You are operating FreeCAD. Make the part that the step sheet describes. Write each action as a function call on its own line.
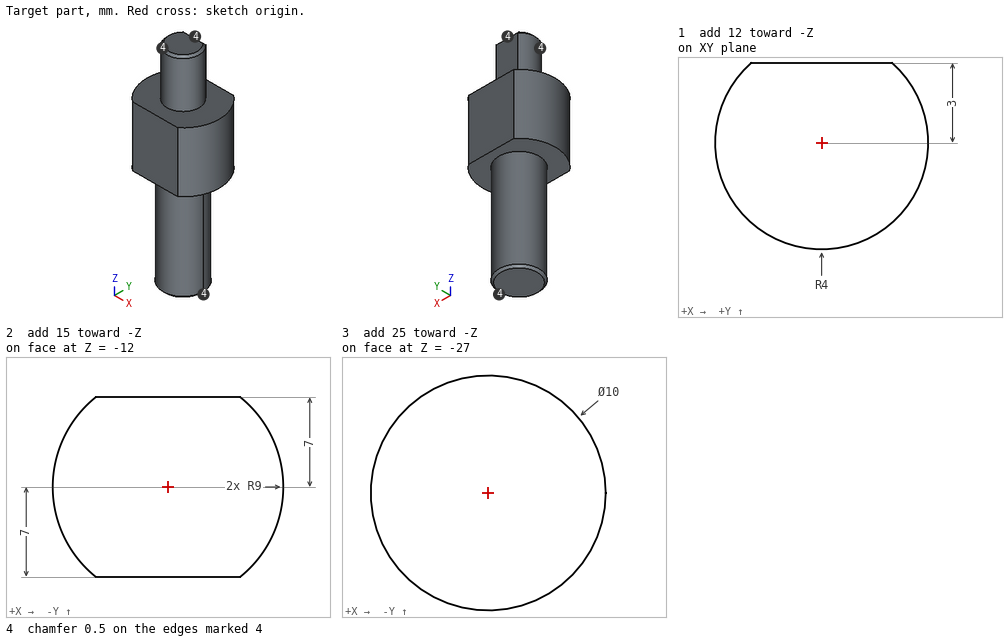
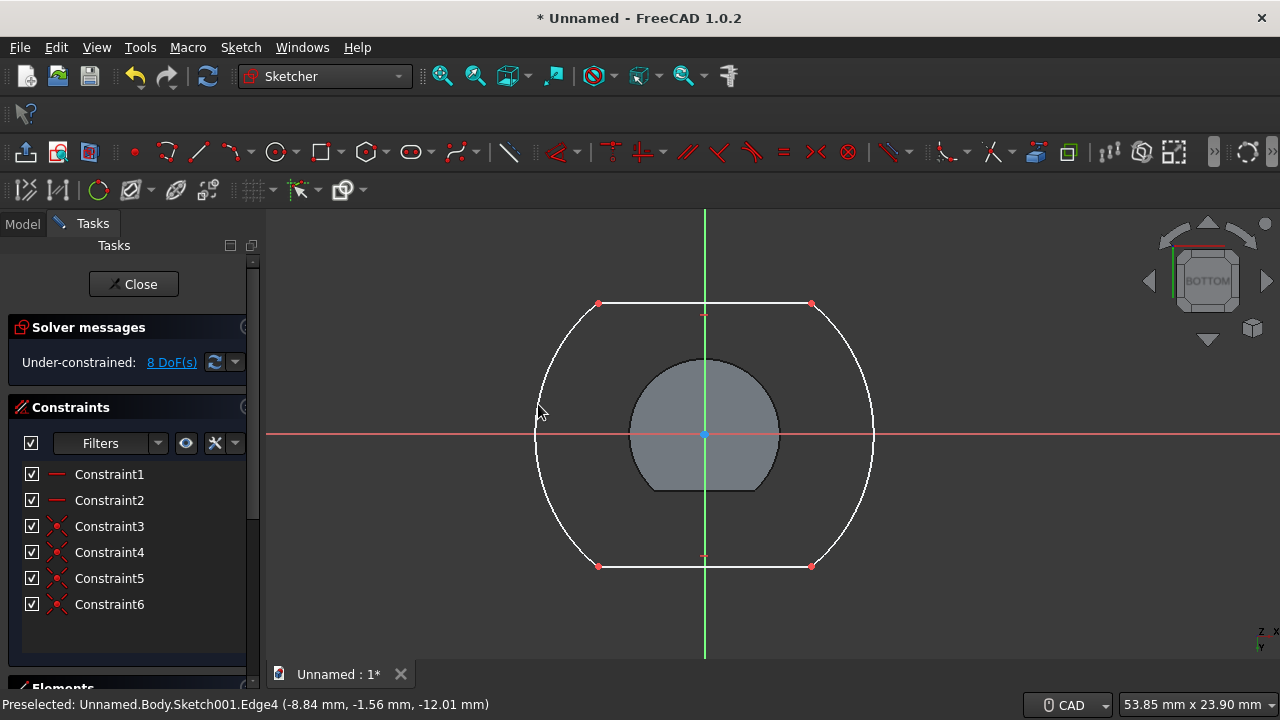
click(863, 494)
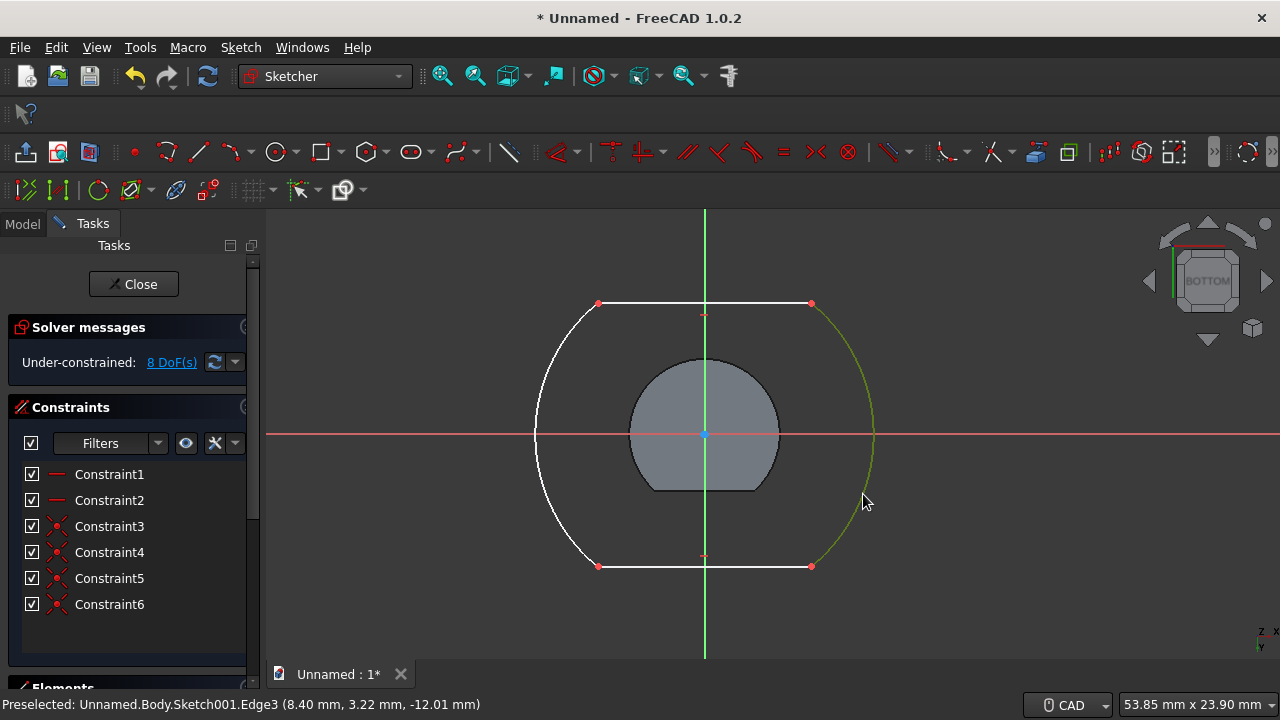
click(546, 376)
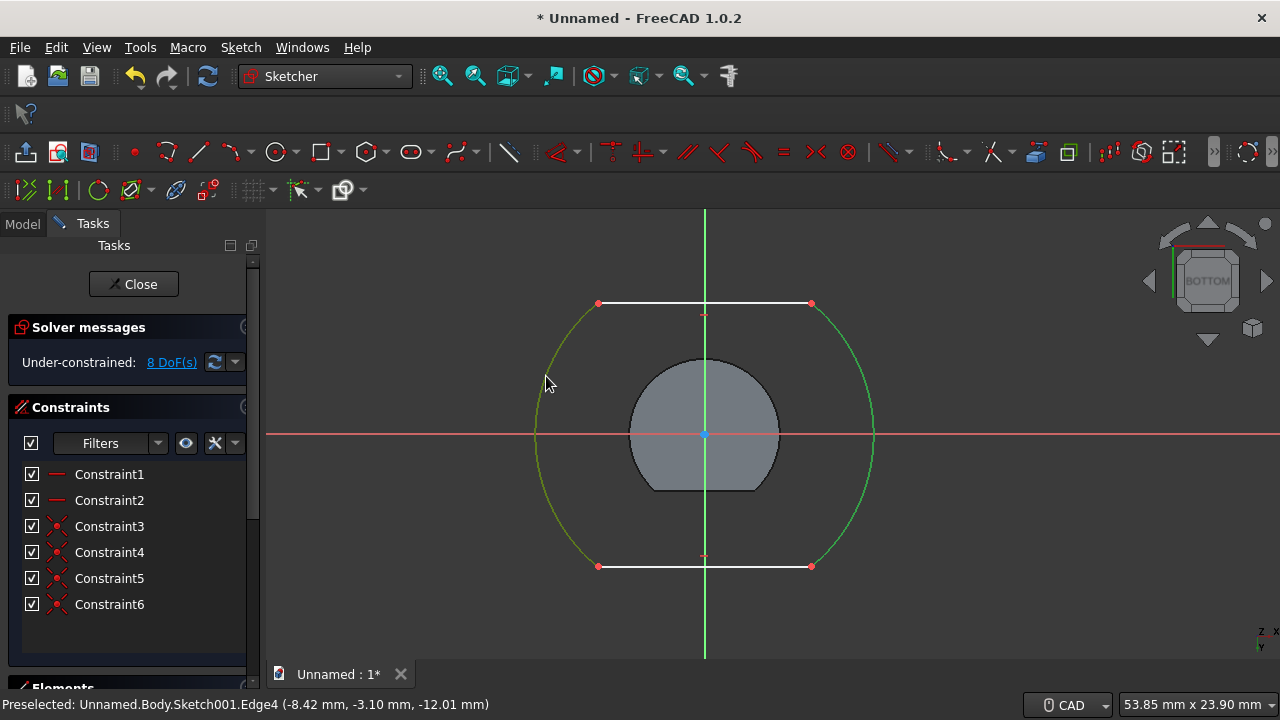
key(c)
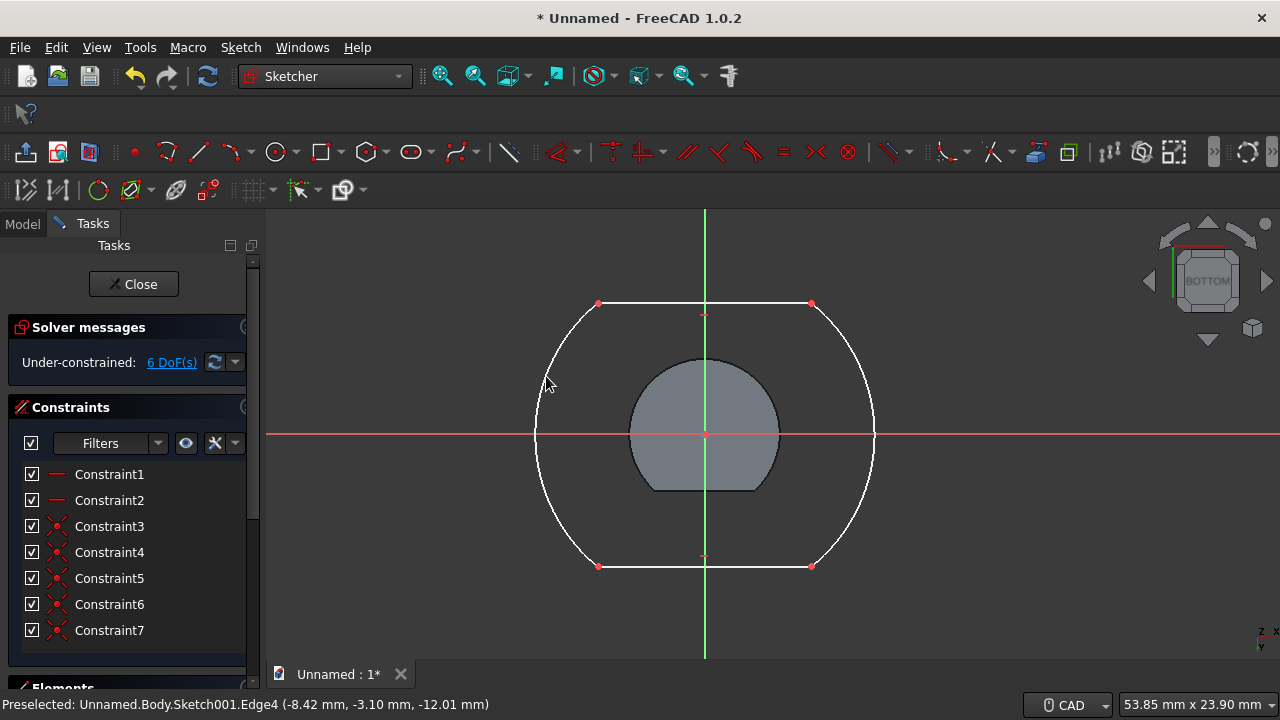
drag(695, 424, 716, 445)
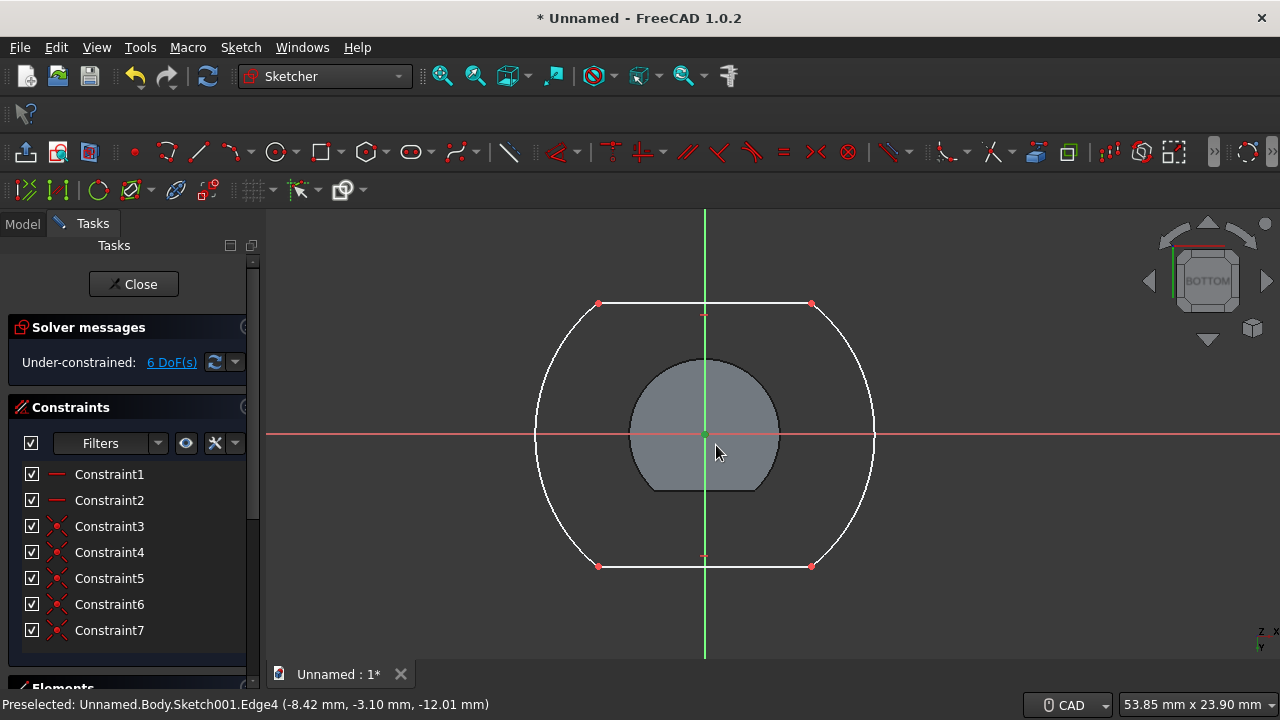
click(612, 152)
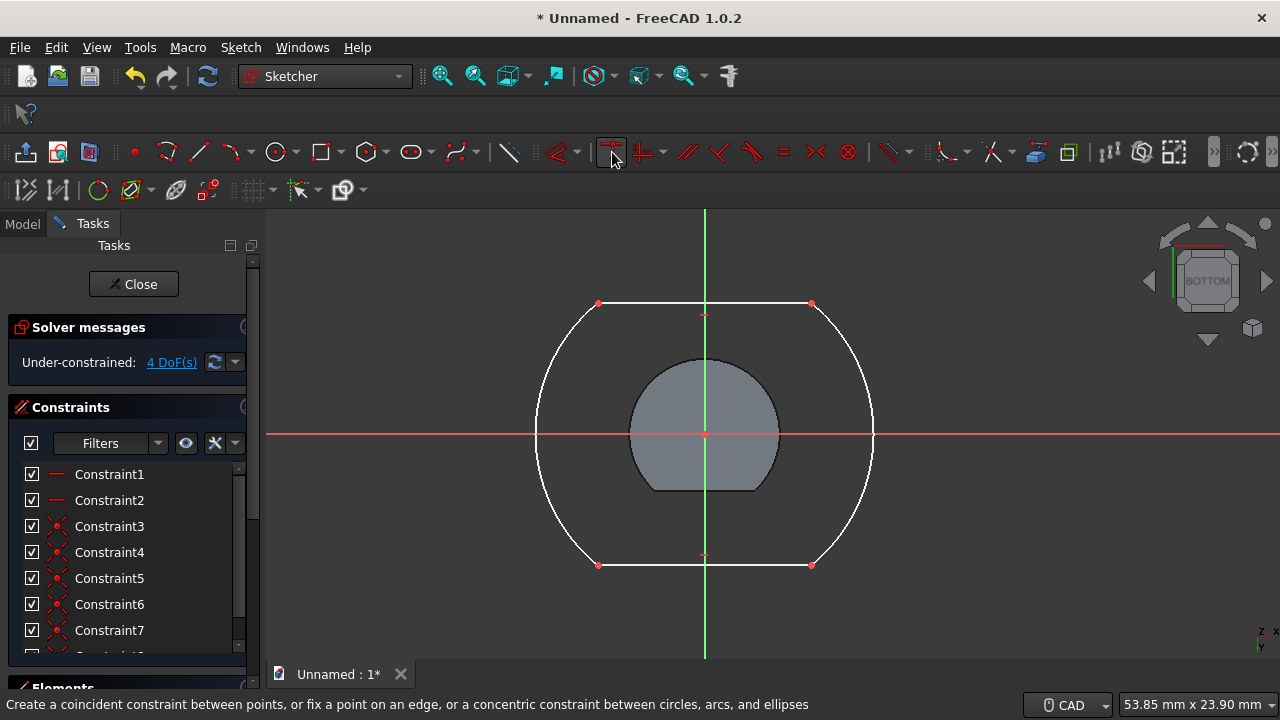
click(863, 493)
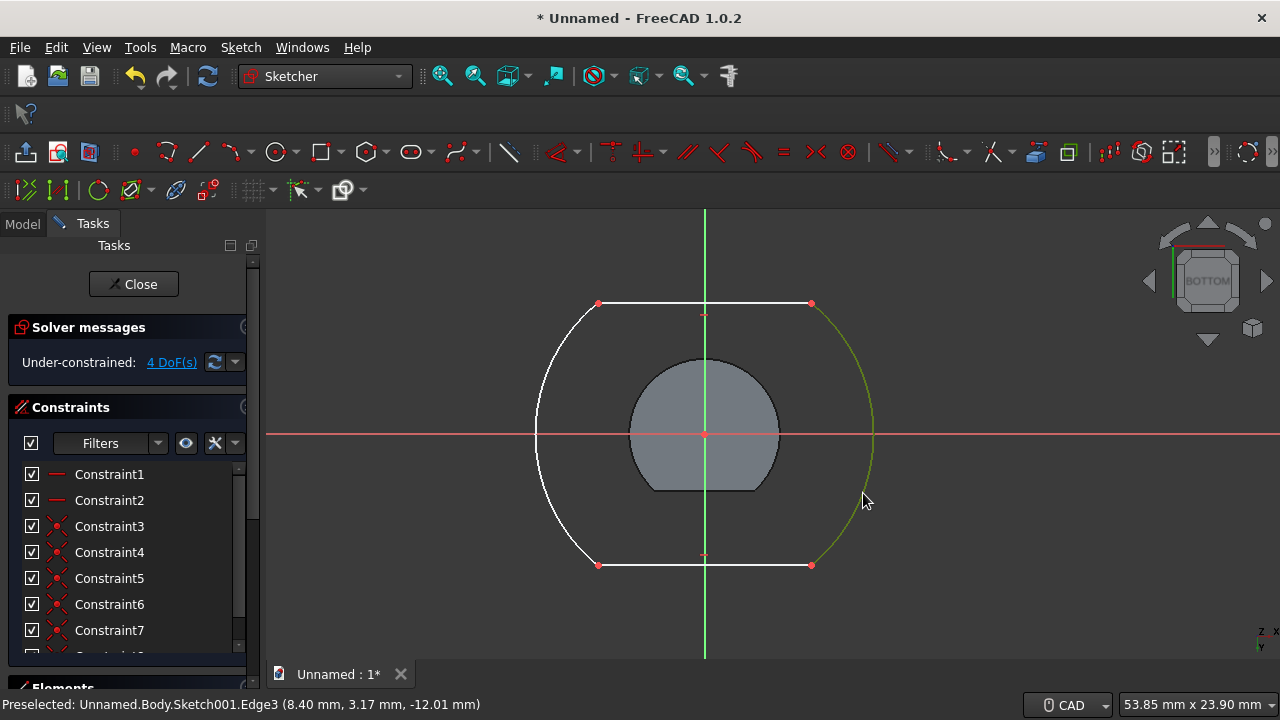
click(546, 375)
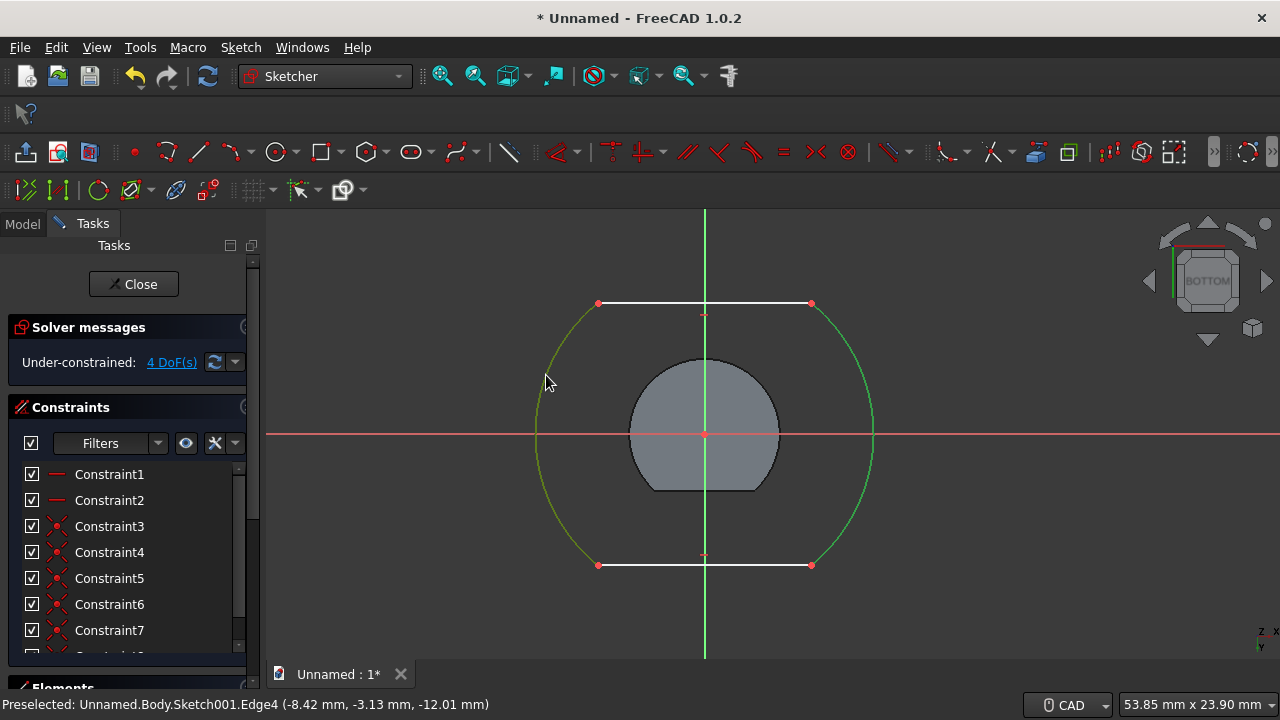
key(e)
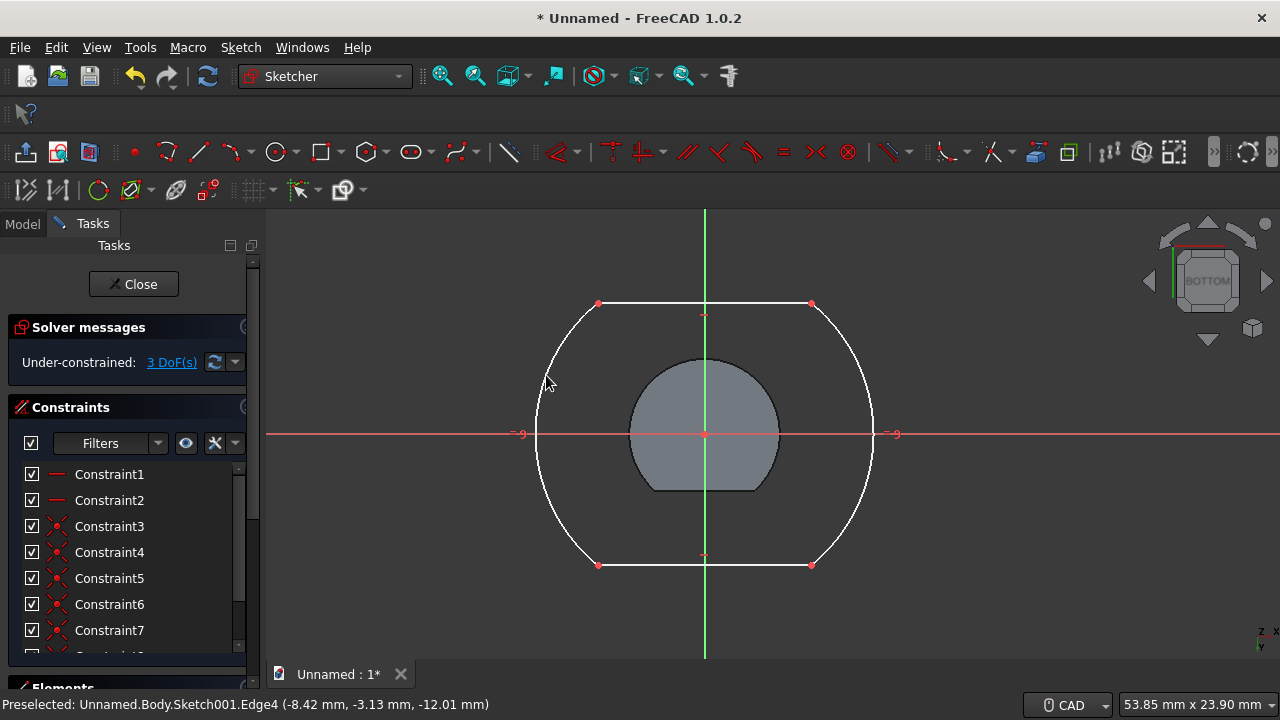
key(d)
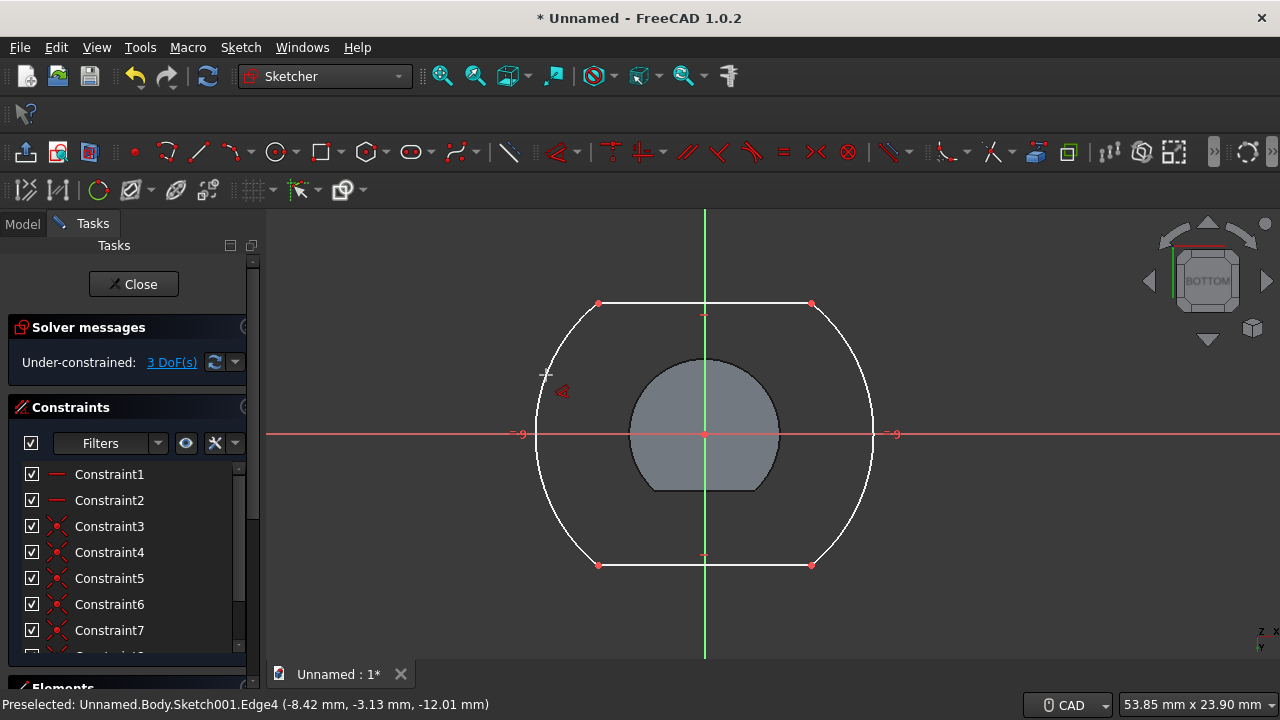
click(863, 493)
click(893, 504)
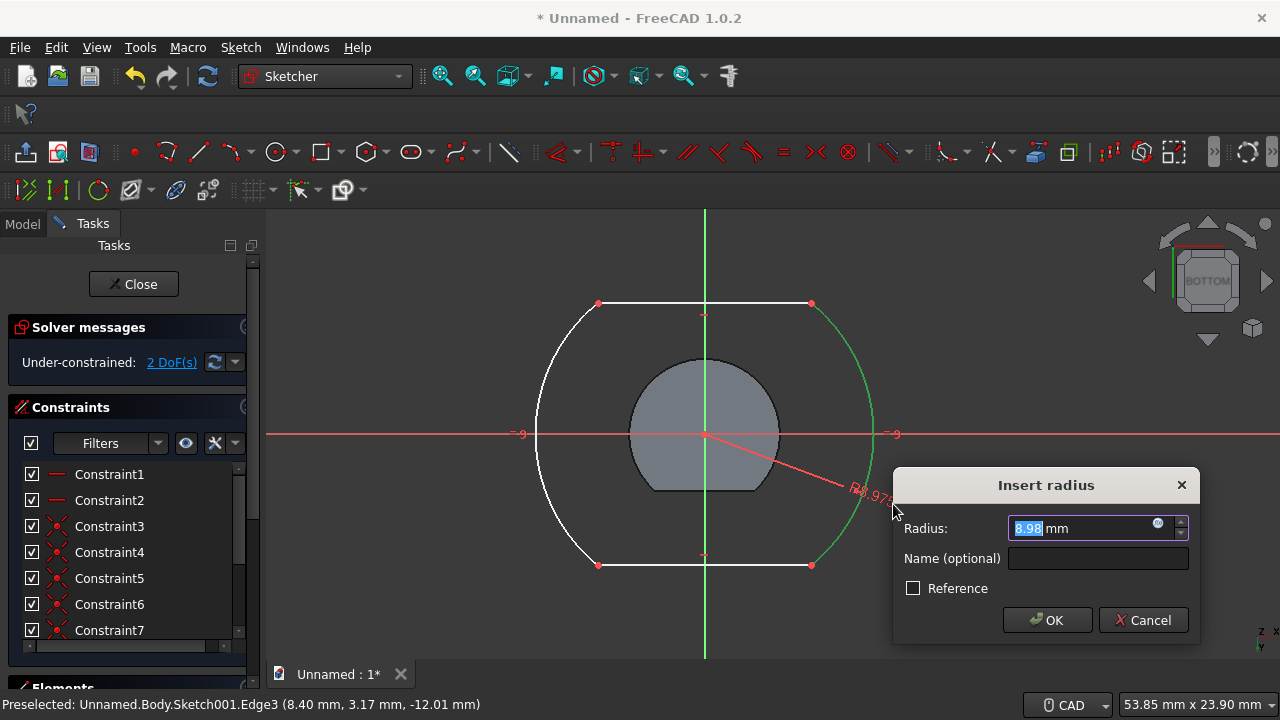
text(9)
key(Return)